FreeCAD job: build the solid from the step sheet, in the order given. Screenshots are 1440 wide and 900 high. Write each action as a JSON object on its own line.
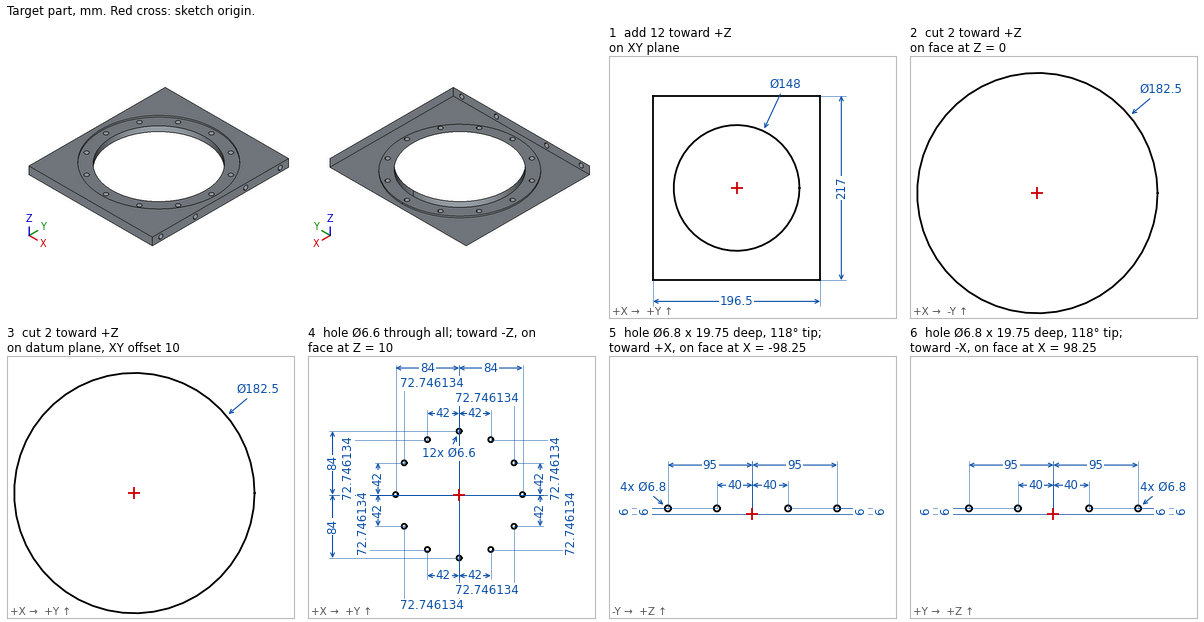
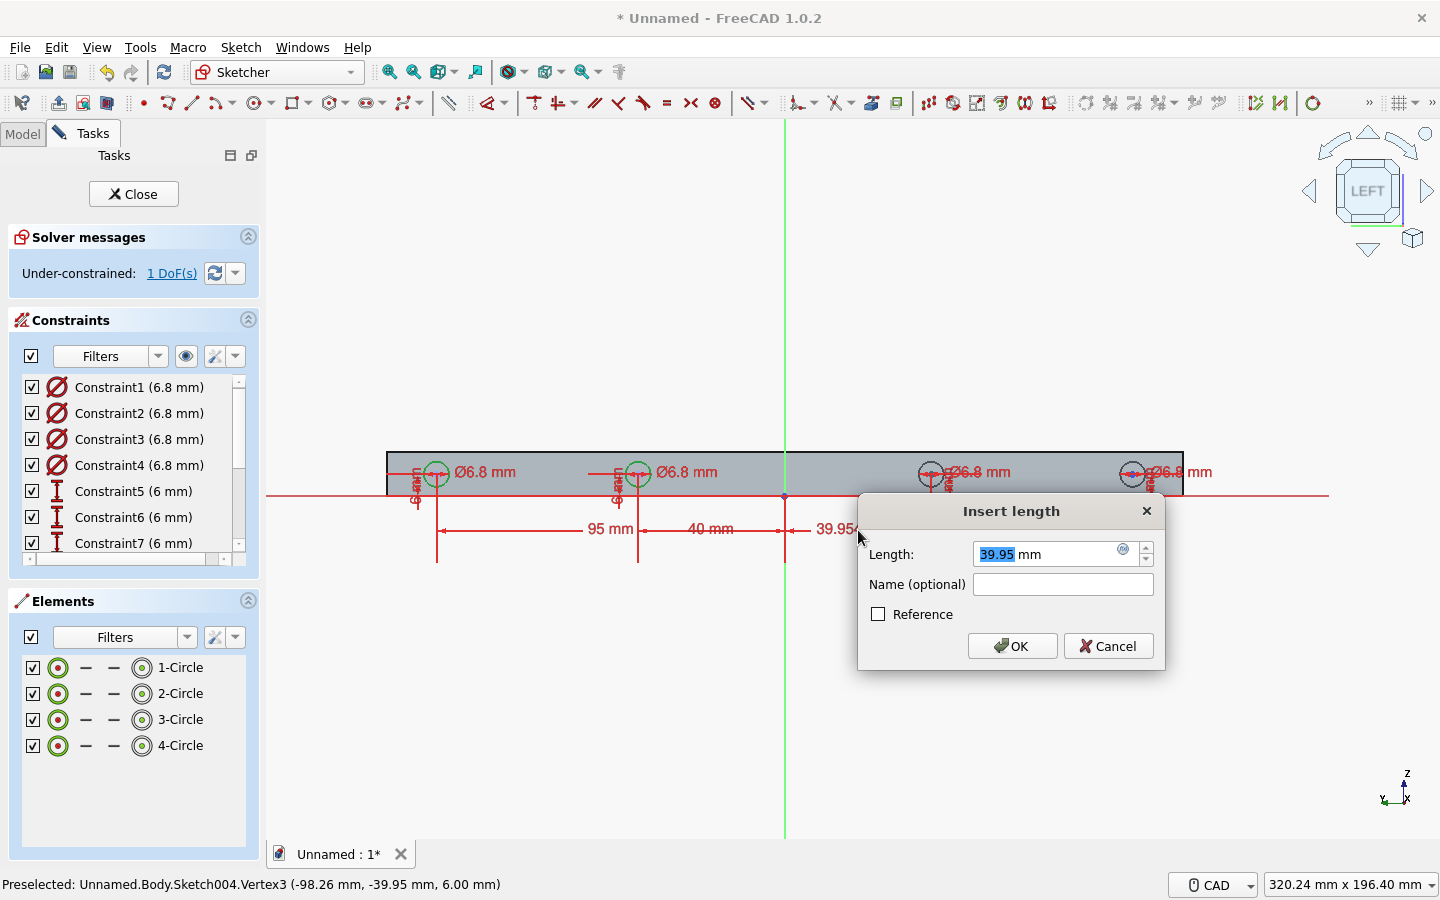
{"action": "type", "text": "40"}
{"action": "key", "text": "Return"}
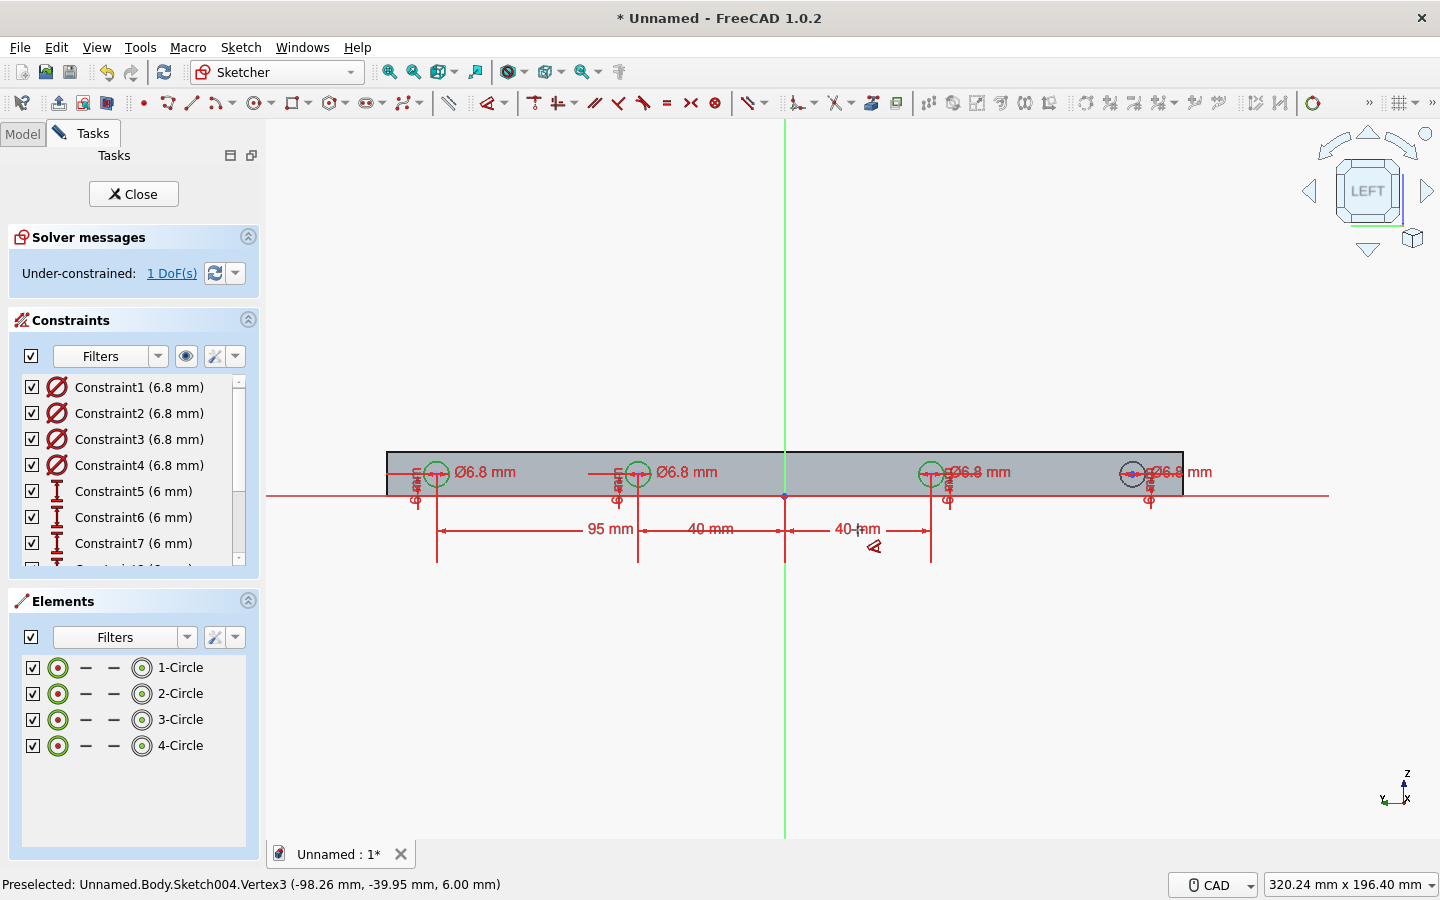
{"action": "left_click", "coordinate": [1133, 474]}
{"action": "left_click", "coordinate": [959, 530]}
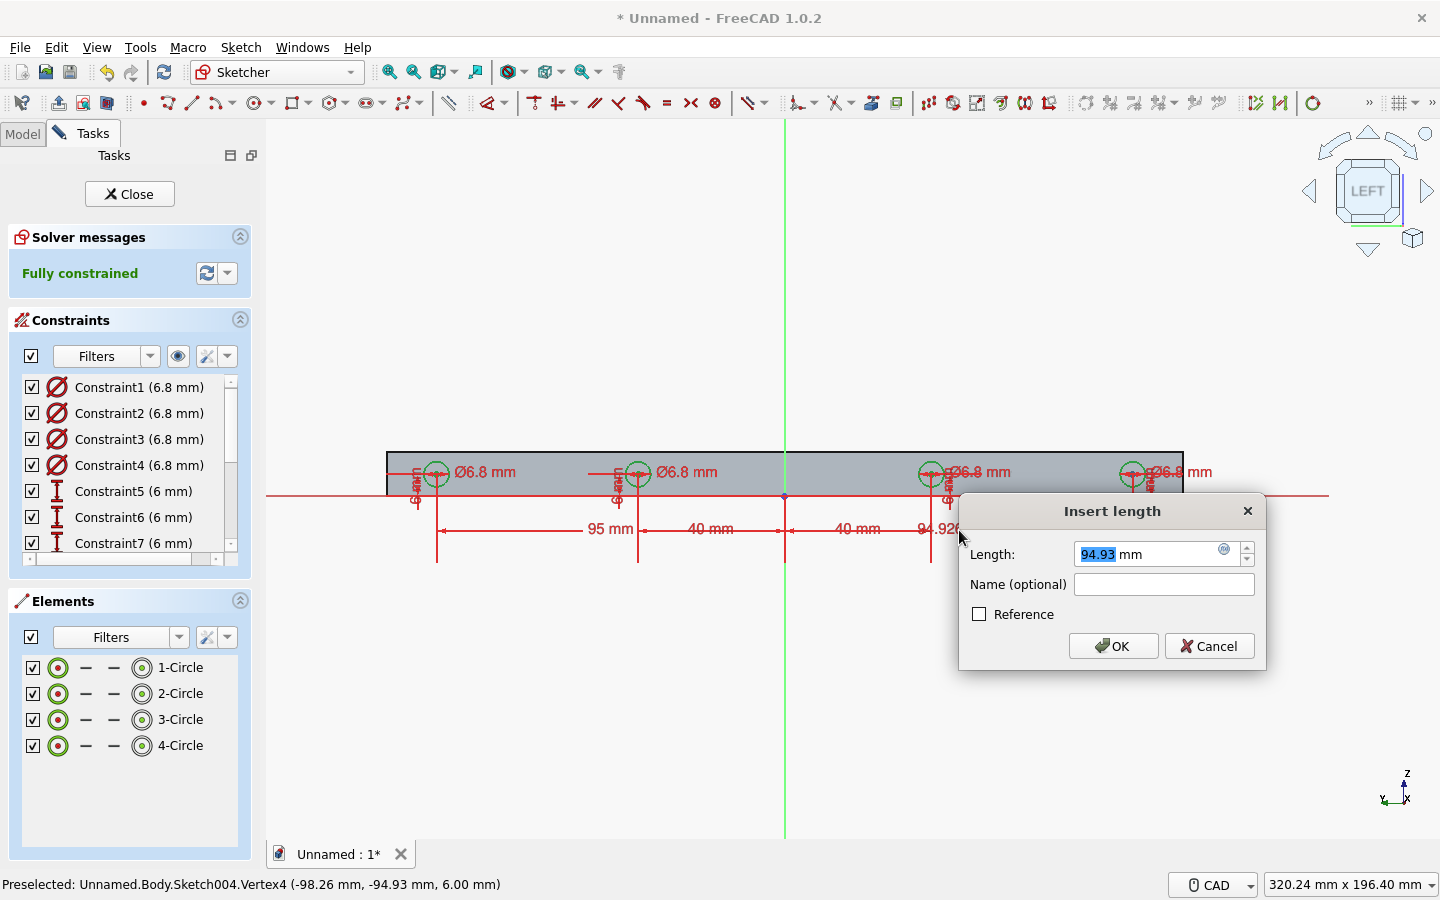
{"action": "type", "text": "95"}
{"action": "key", "text": "Return"}
{"action": "key", "text": "Escape"}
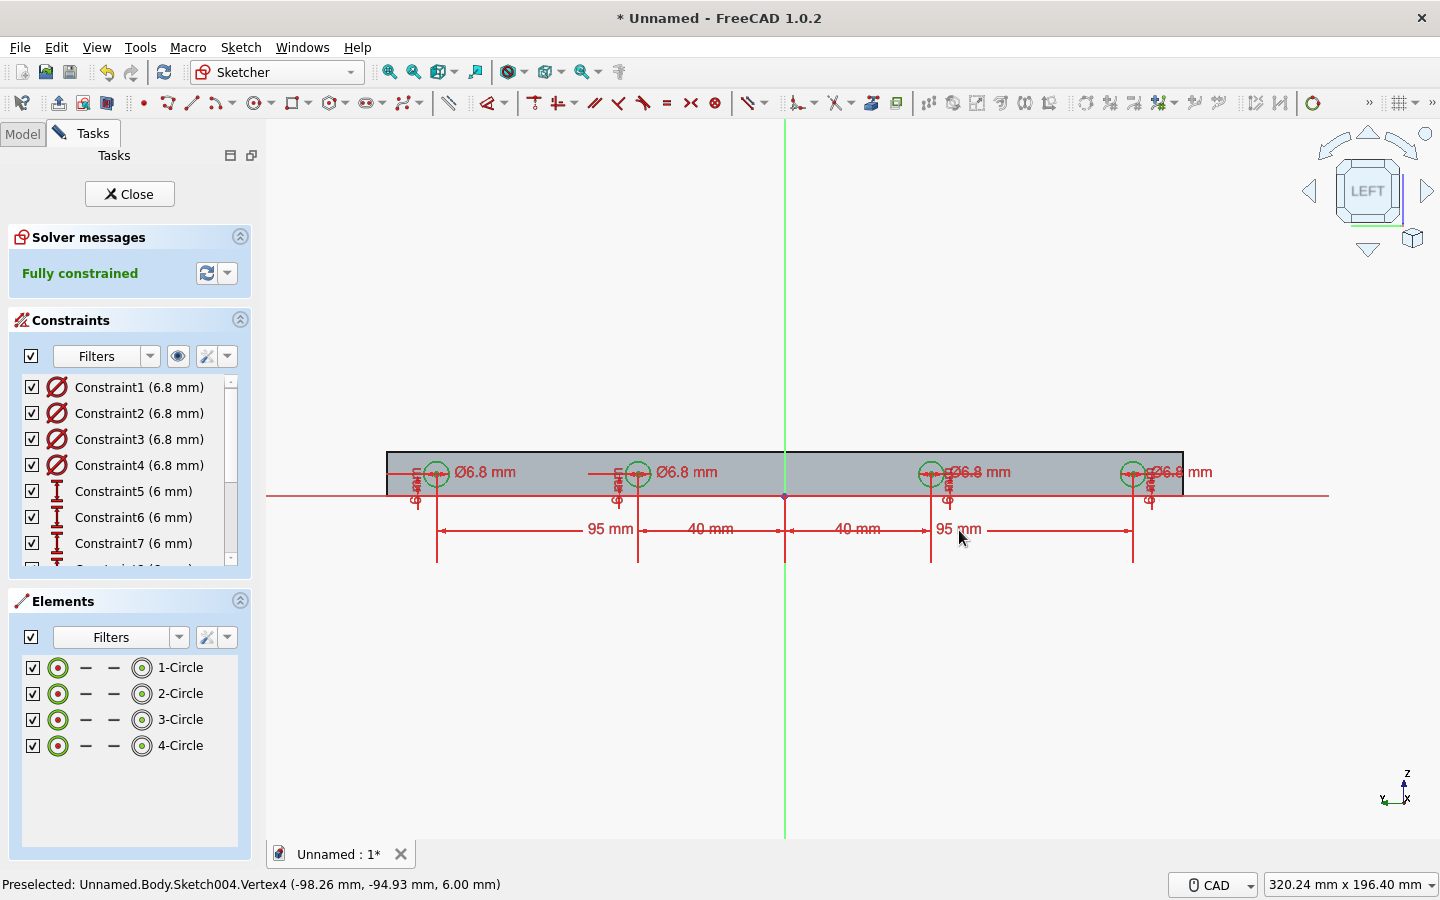
{"action": "left_click", "coordinate": [130, 194]}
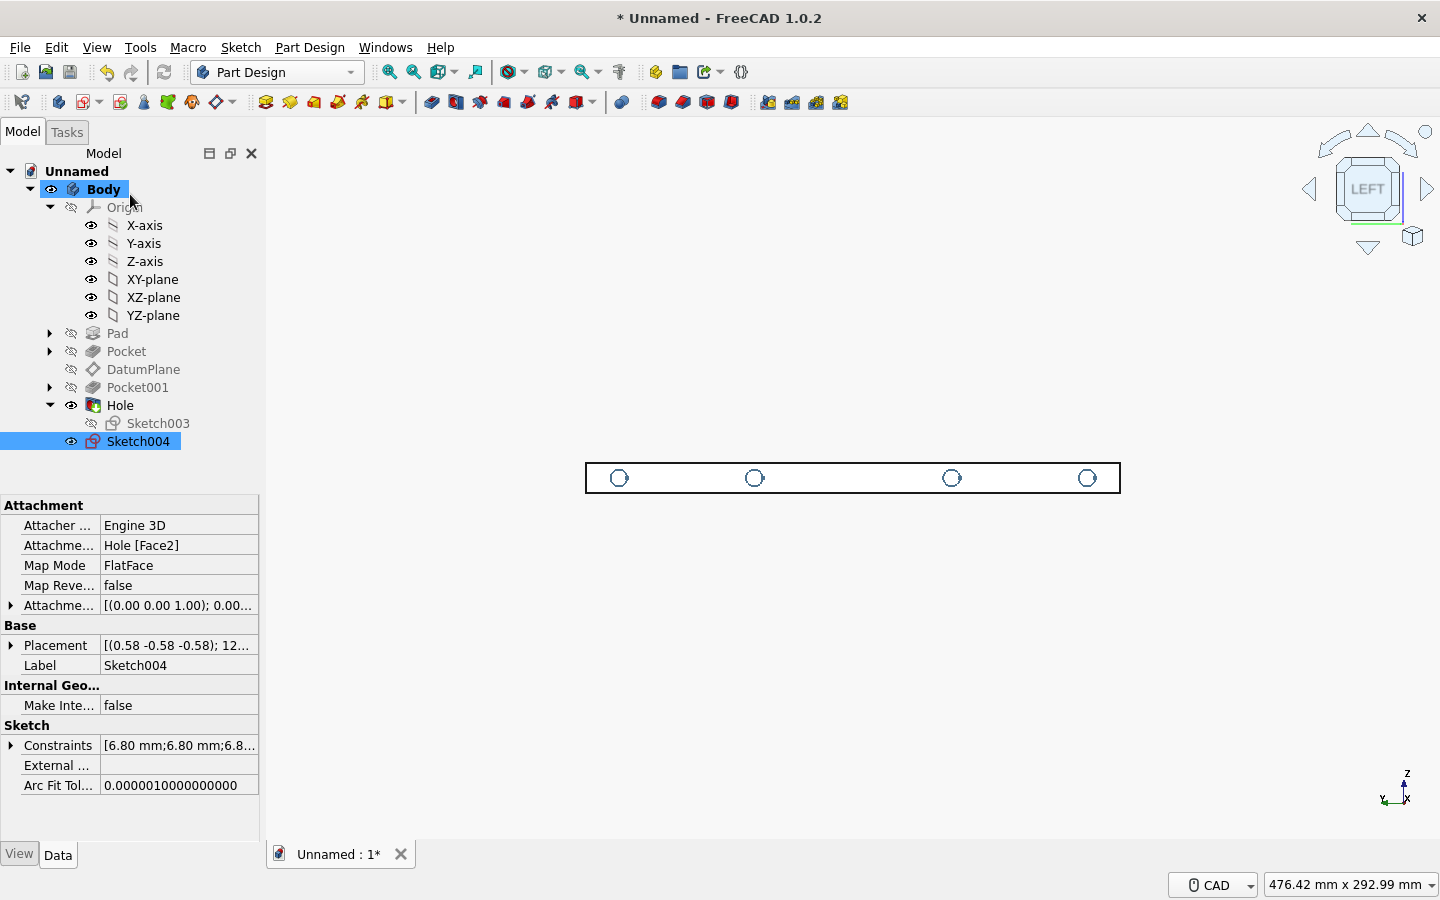
{"action": "left_click", "coordinate": [456, 102]}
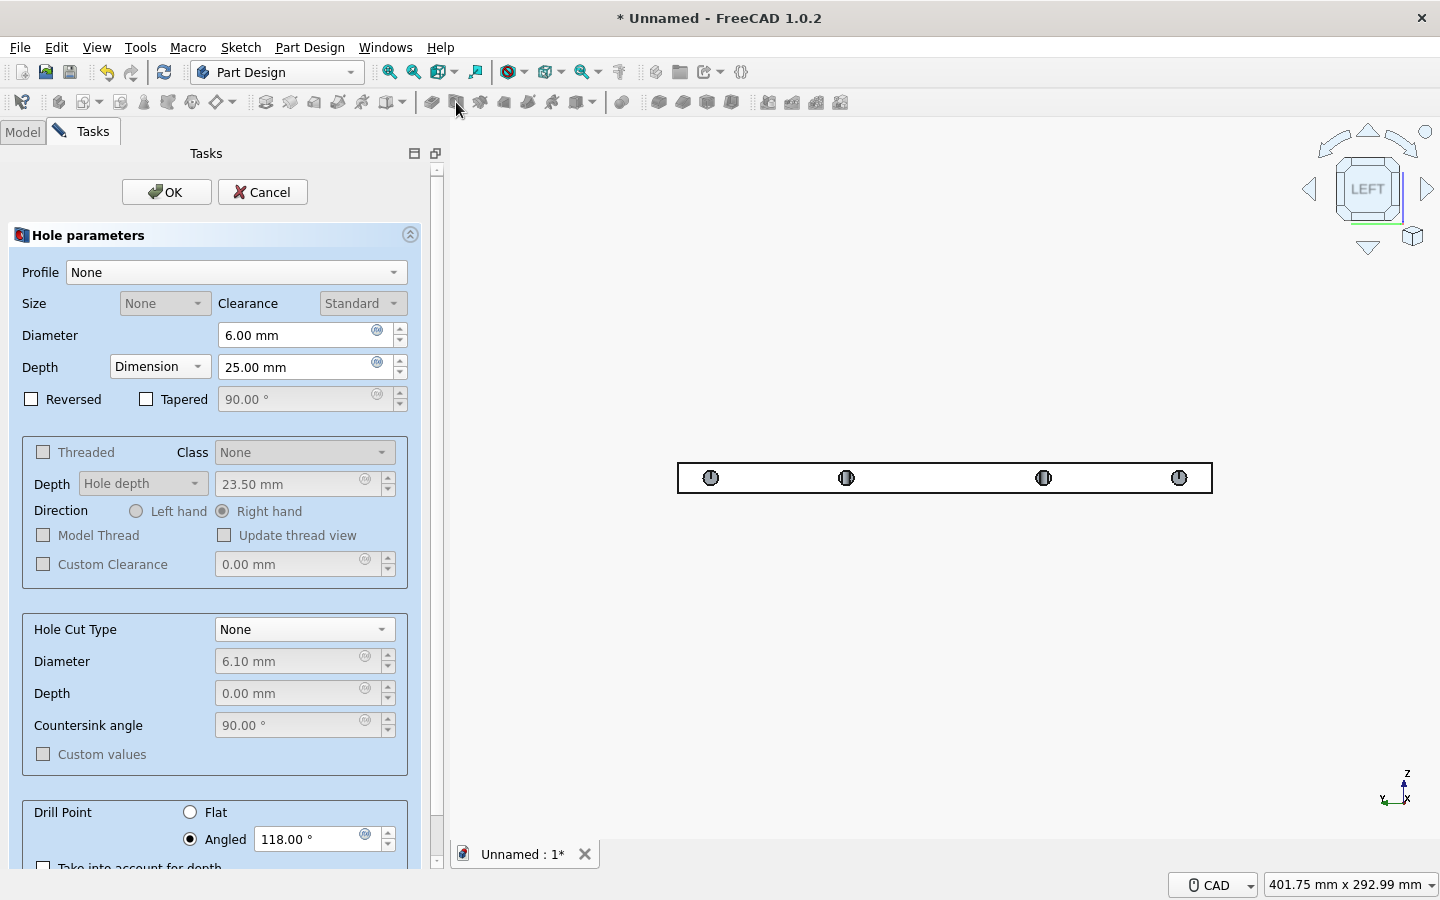
{"action": "triple_click", "coordinate": [305, 335]}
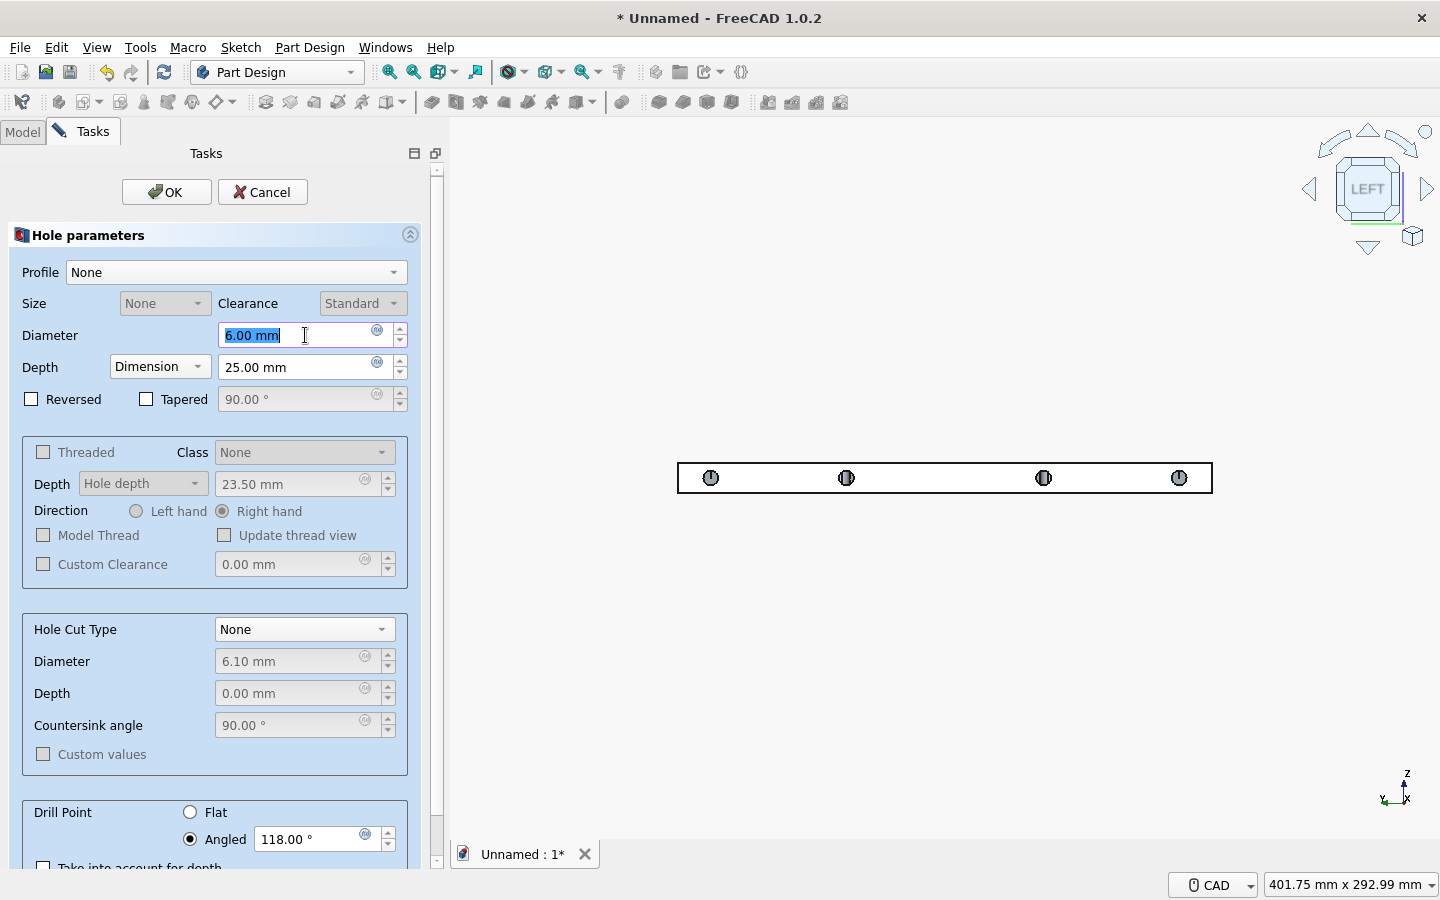
{"action": "type", "text": "6.8"}
{"action": "key", "text": "Tab"}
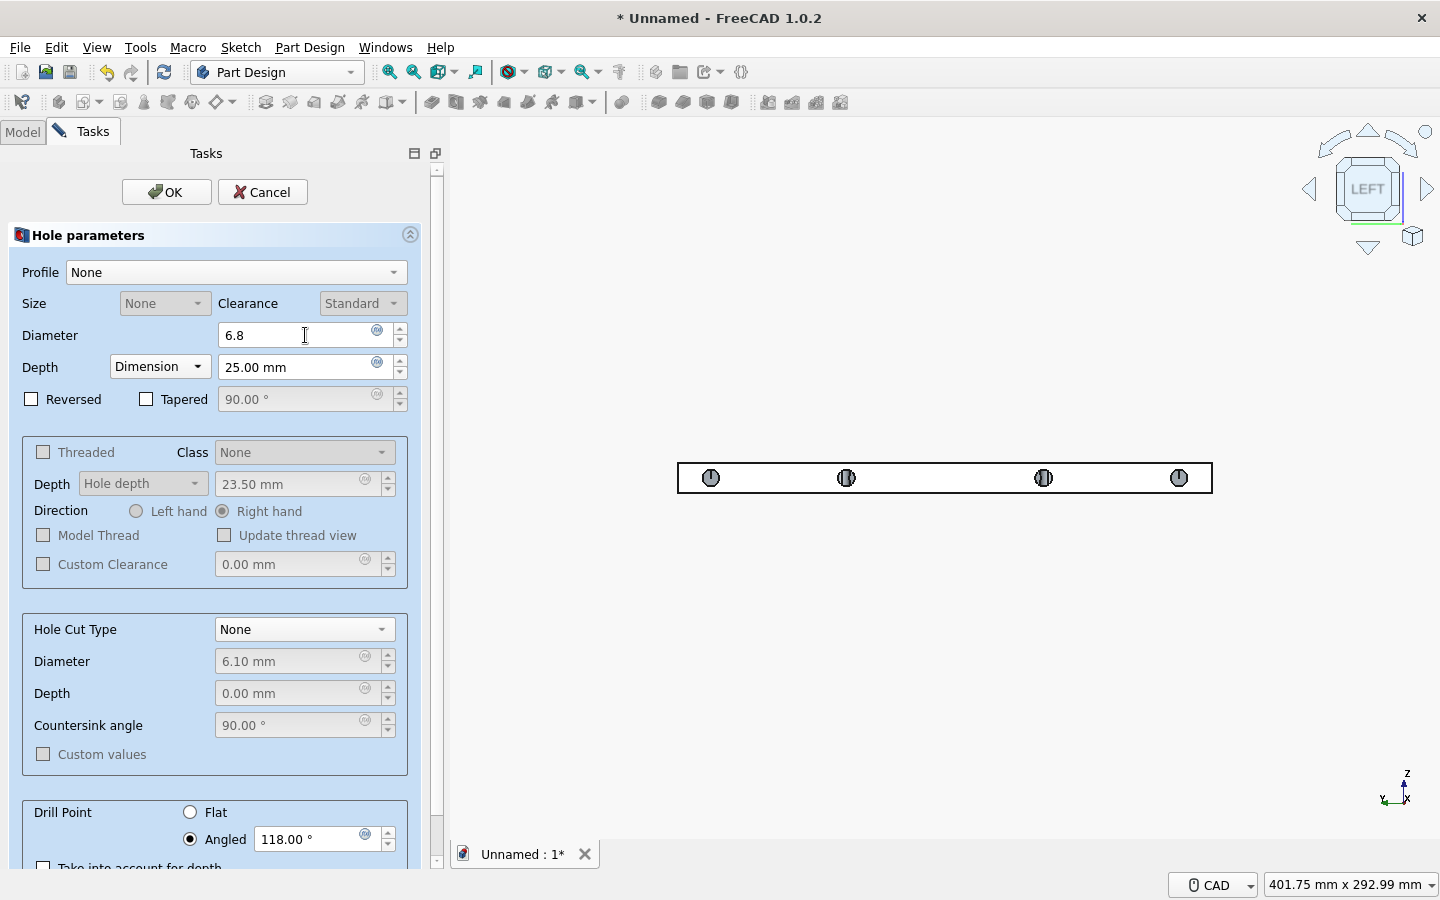
{"action": "triple_click", "coordinate": [305, 367]}